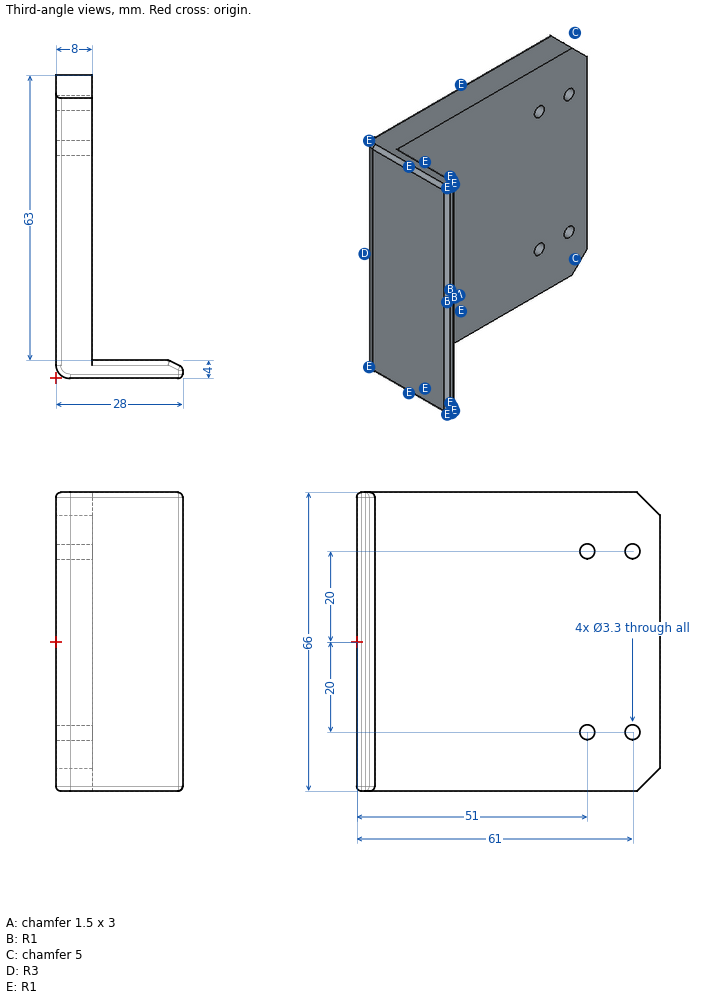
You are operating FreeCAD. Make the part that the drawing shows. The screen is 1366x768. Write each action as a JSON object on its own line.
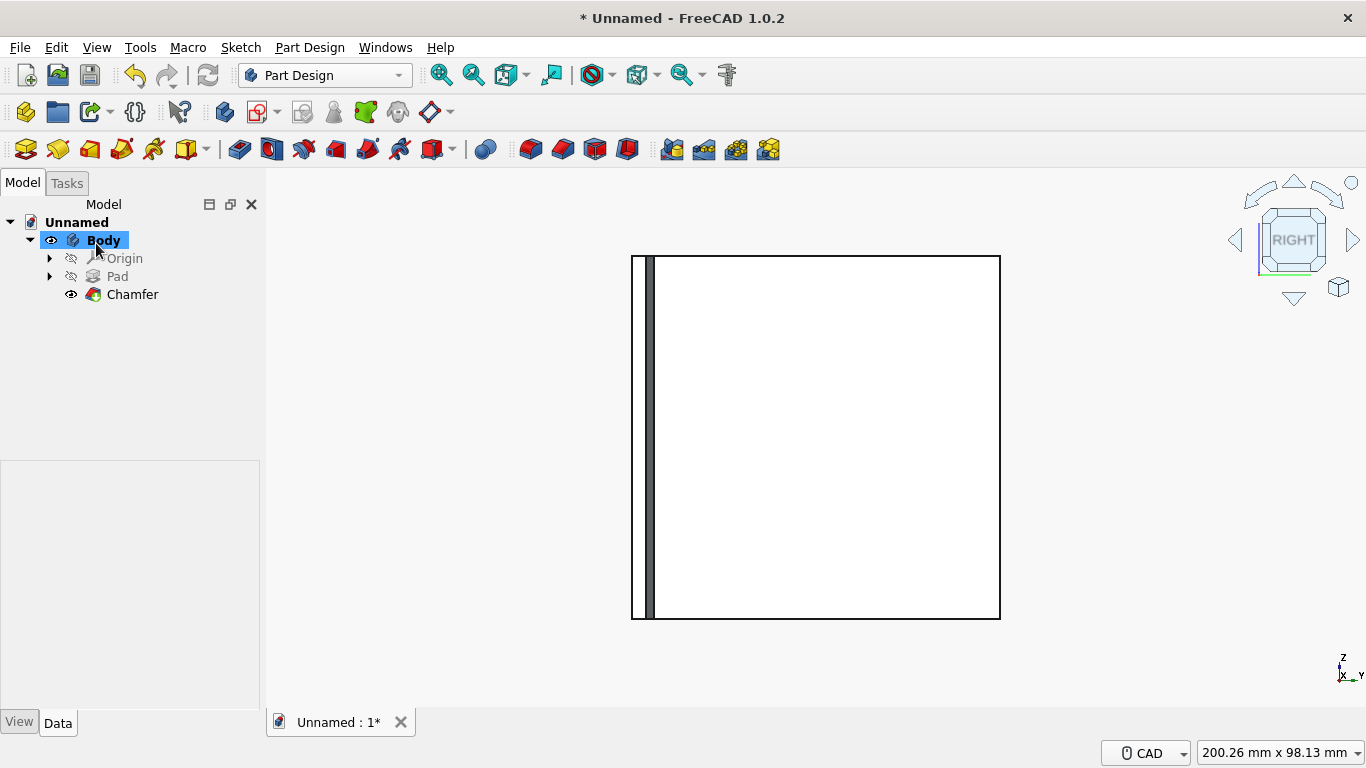
{"action": "left_click", "coordinate": [632, 436]}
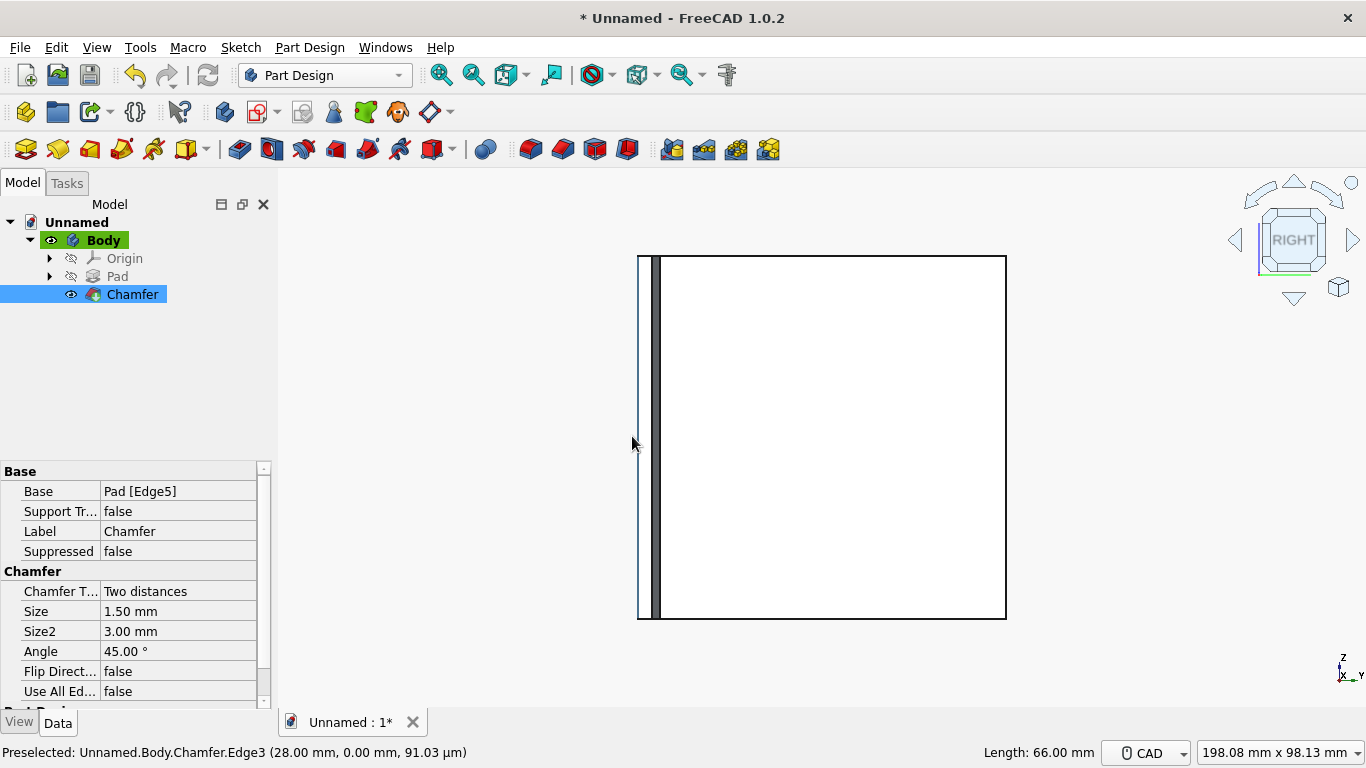
{"action": "left_click", "coordinate": [652, 436], "text": "ctrl"}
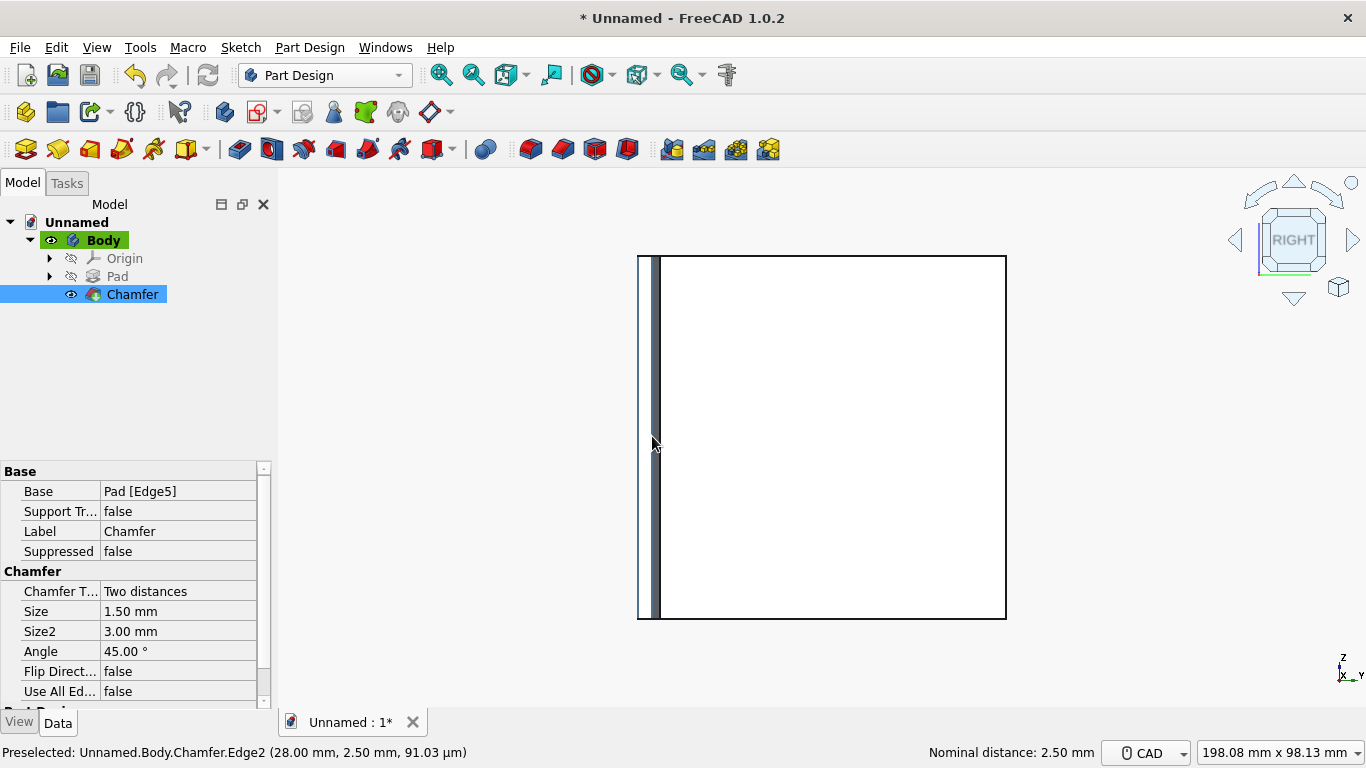
{"action": "key", "text": "0"}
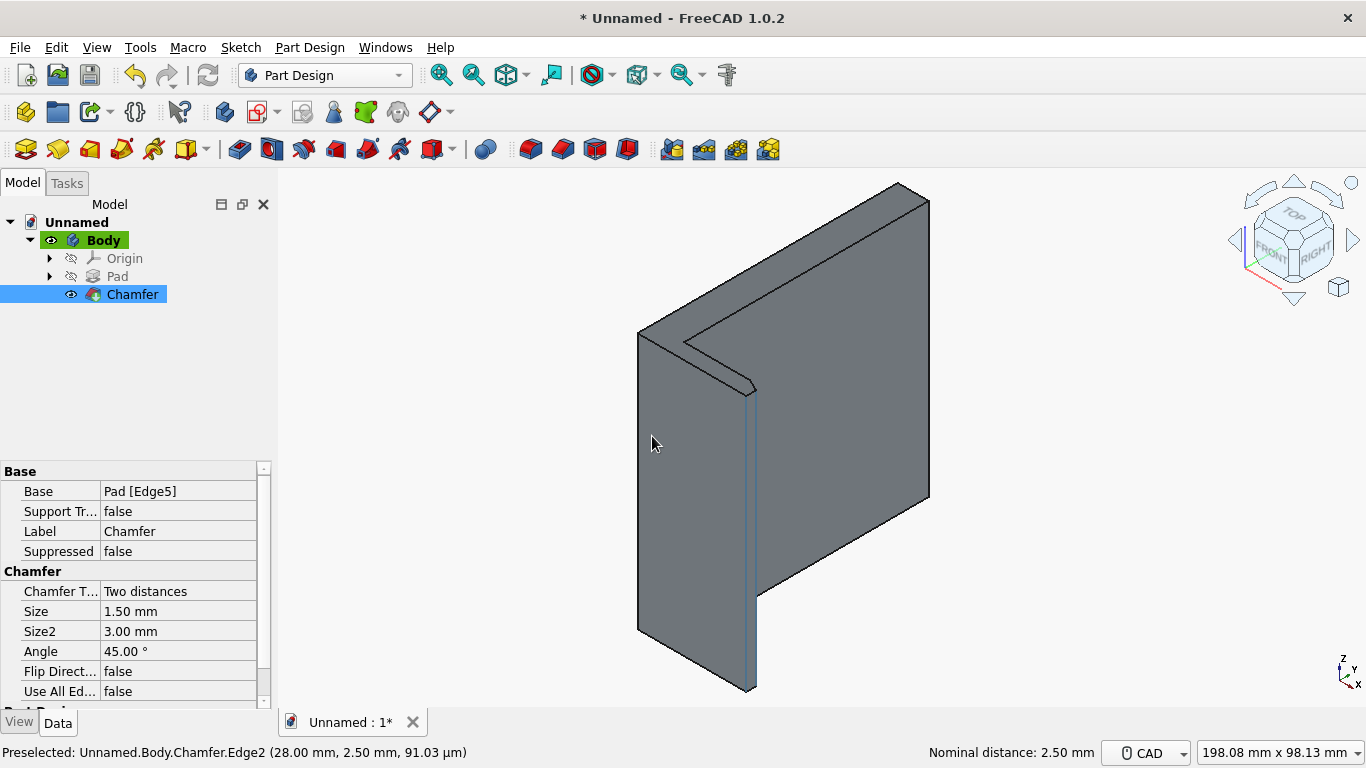
{"action": "key", "text": "2"}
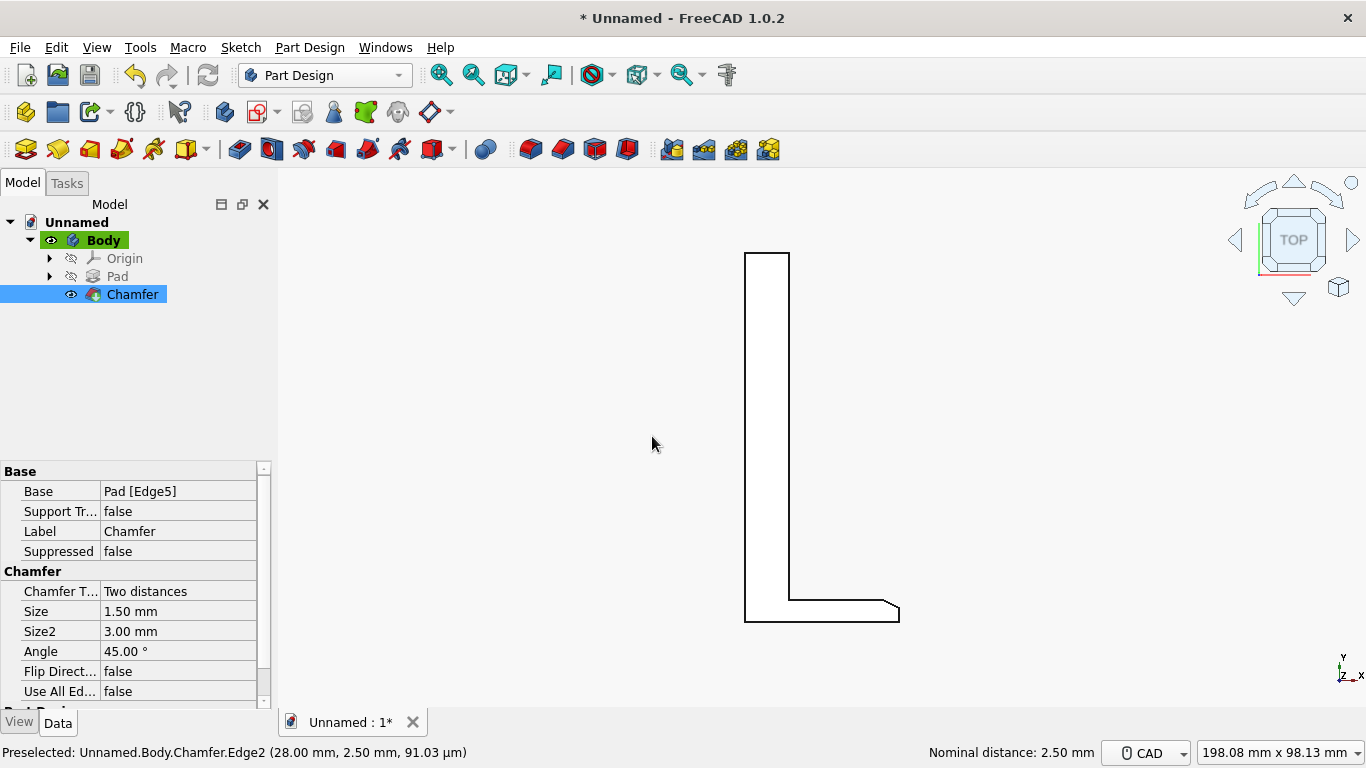
{"action": "key", "text": "1"}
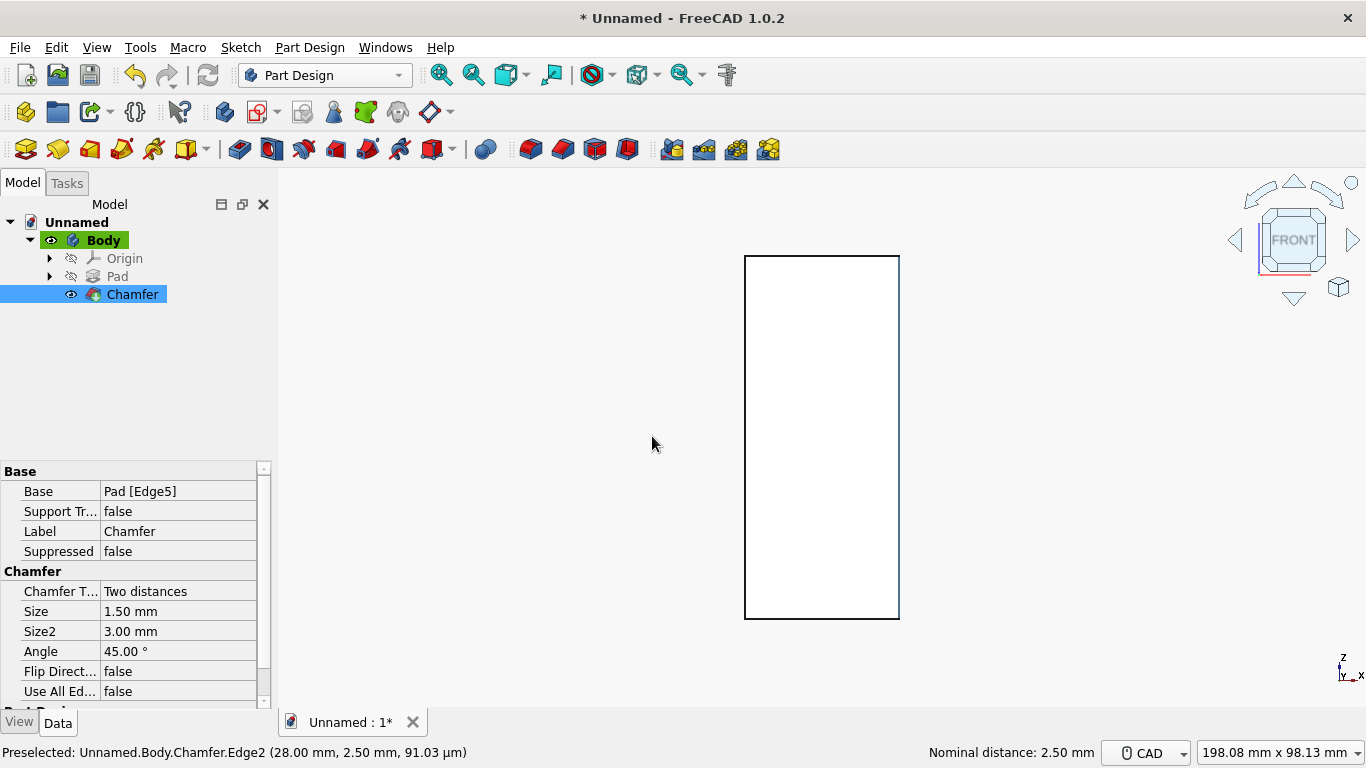
{"action": "key", "text": "3"}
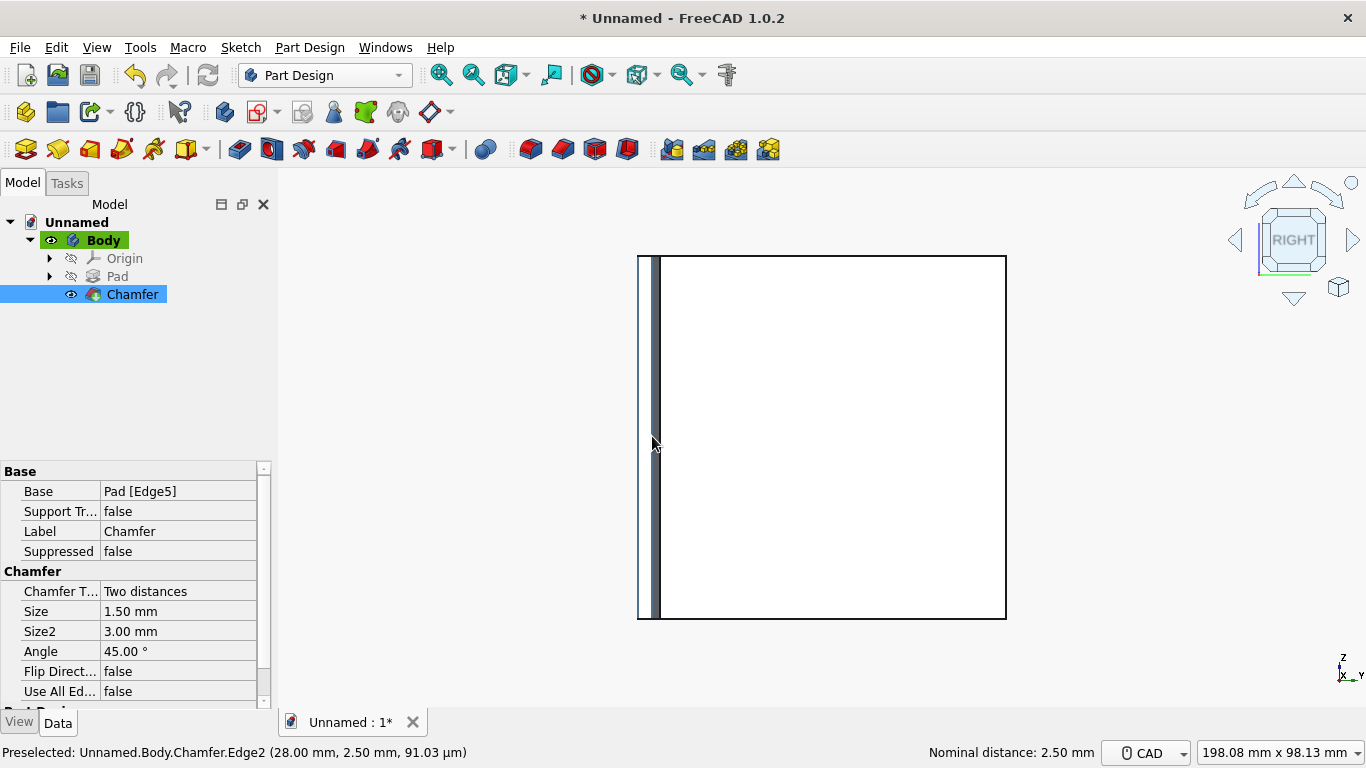
{"action": "key", "text": "5"}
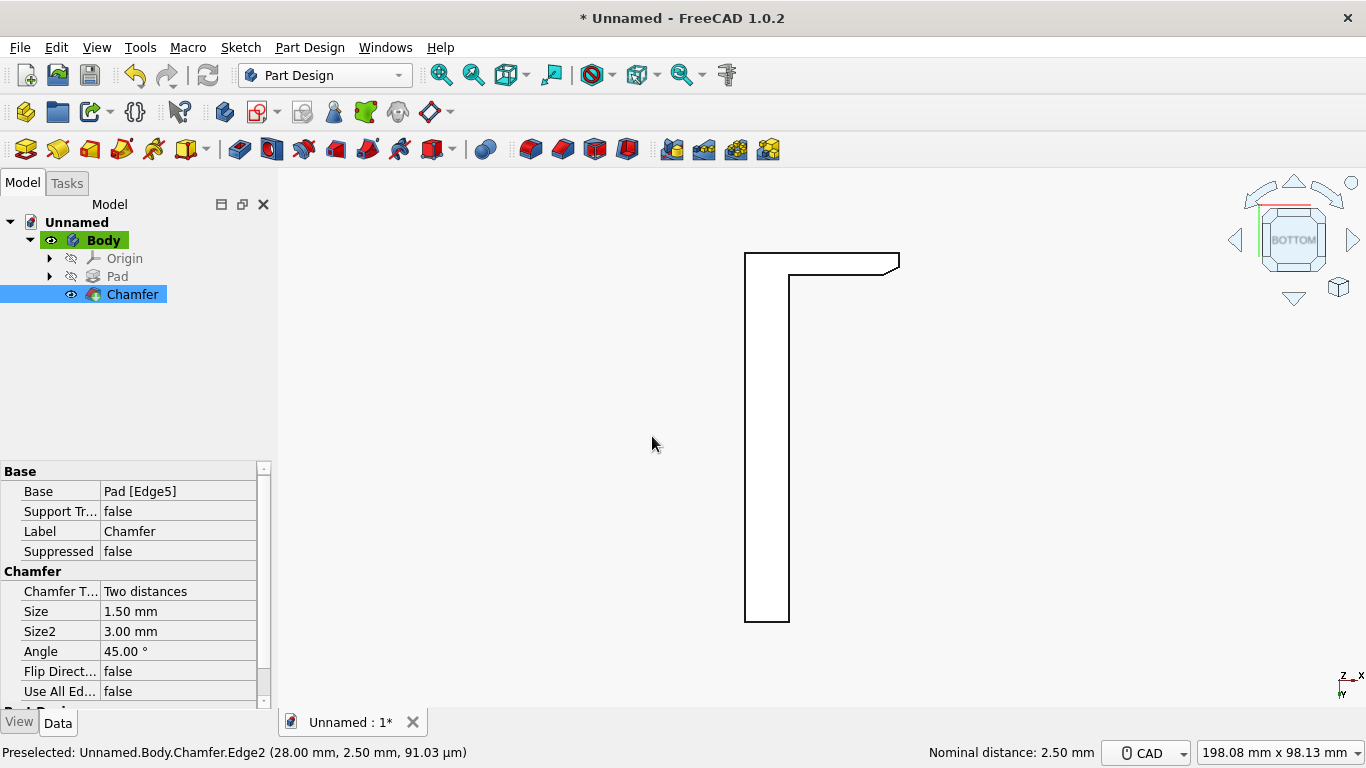
{"action": "key", "text": "4"}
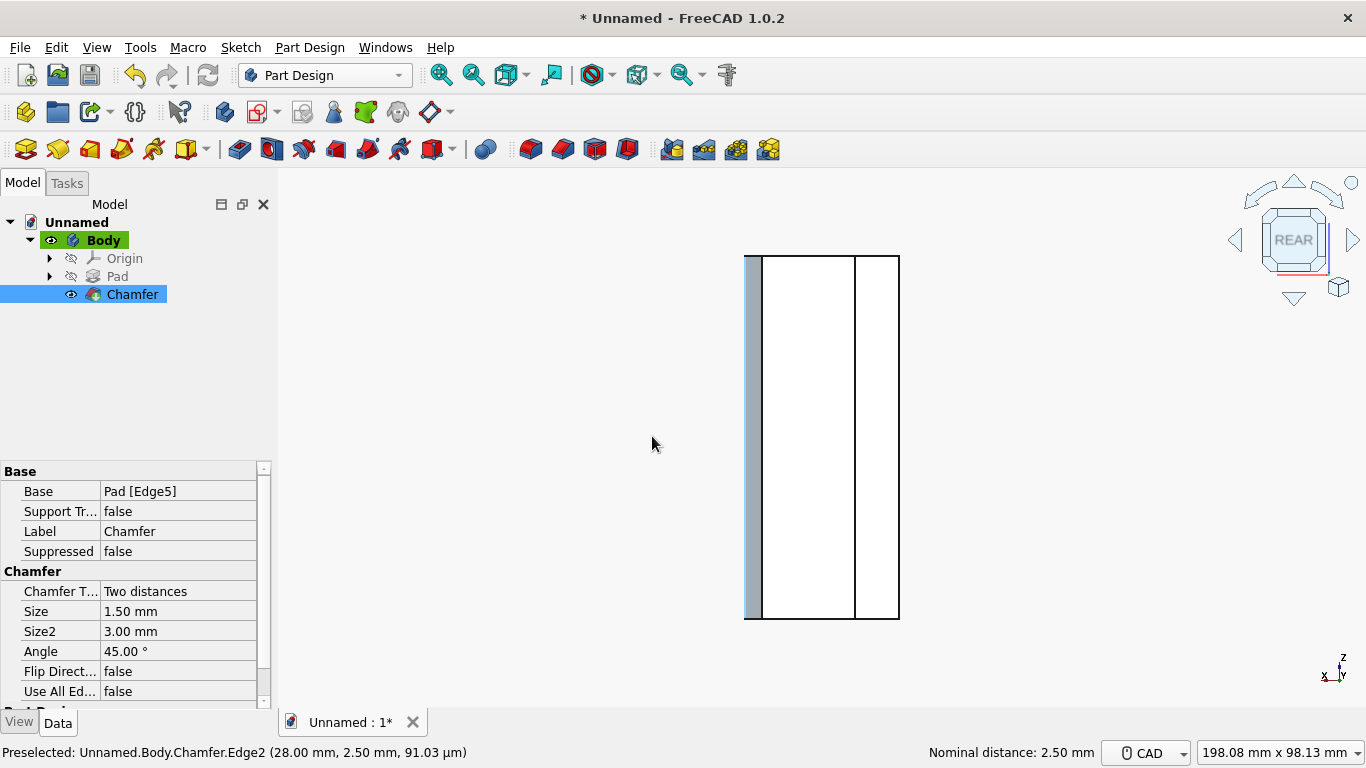
{"action": "left_click", "coordinate": [762, 437], "text": "ctrl"}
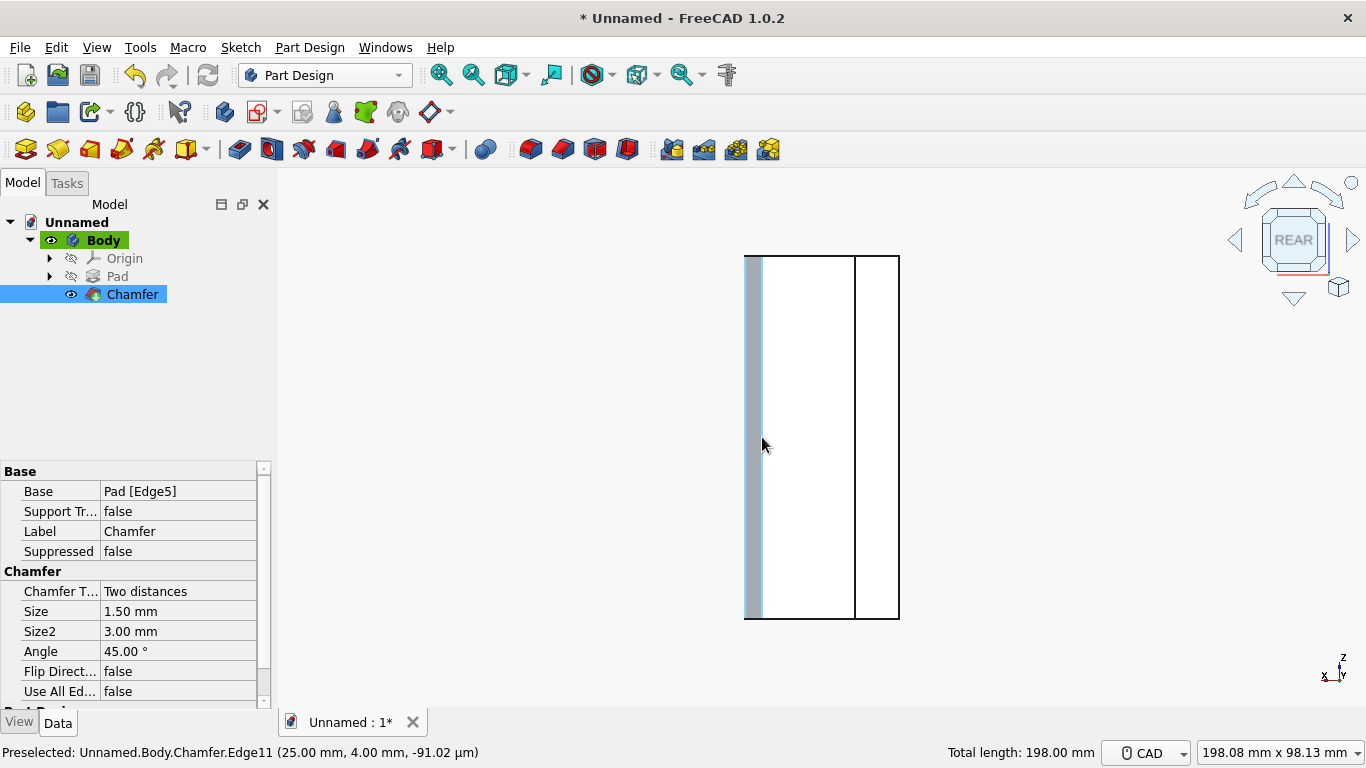
{"action": "left_click", "coordinate": [532, 150]}